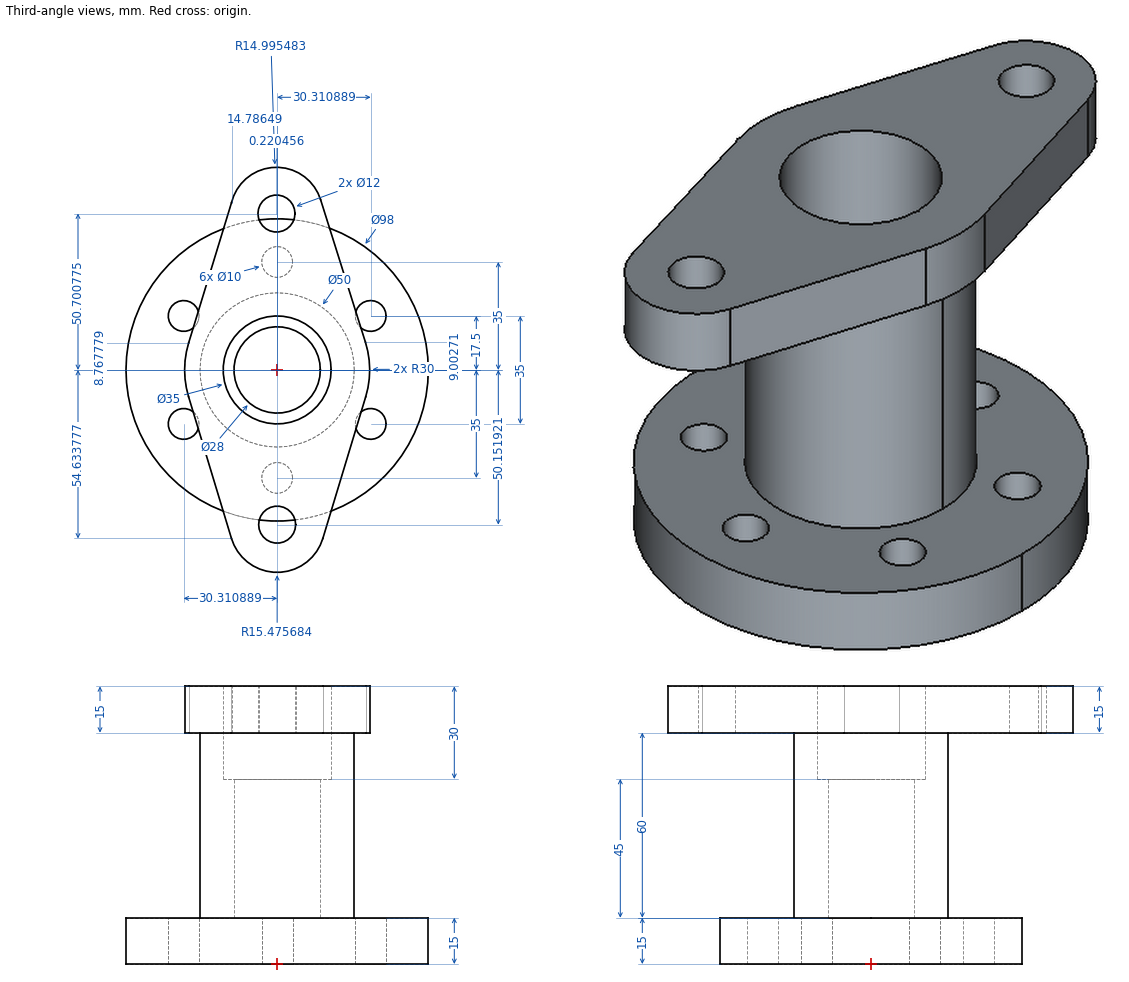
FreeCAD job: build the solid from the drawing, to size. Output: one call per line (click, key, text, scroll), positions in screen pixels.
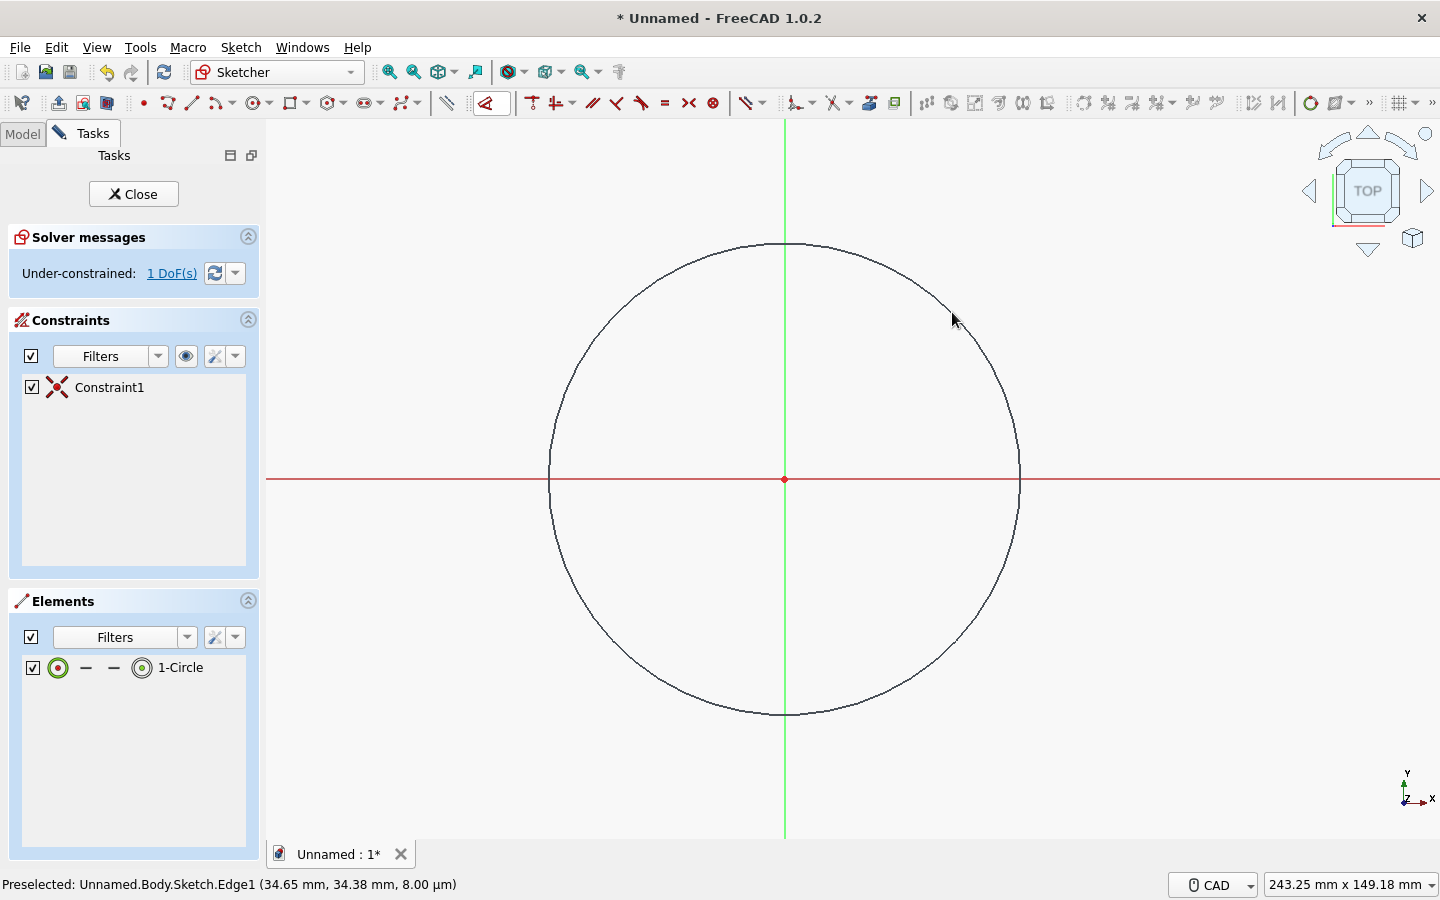
click(951, 312)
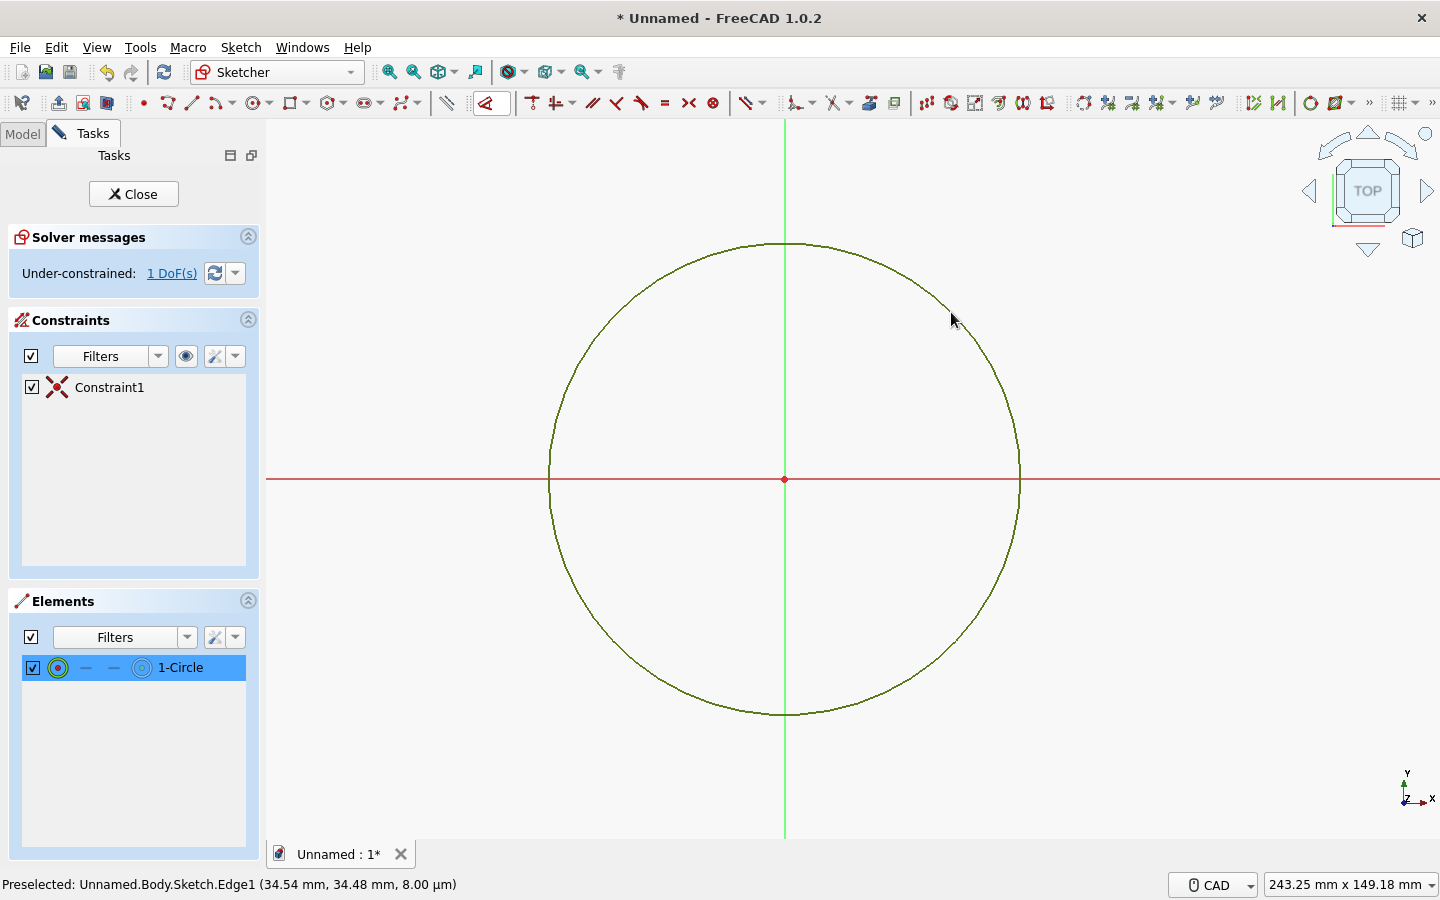
key(k)
key(o)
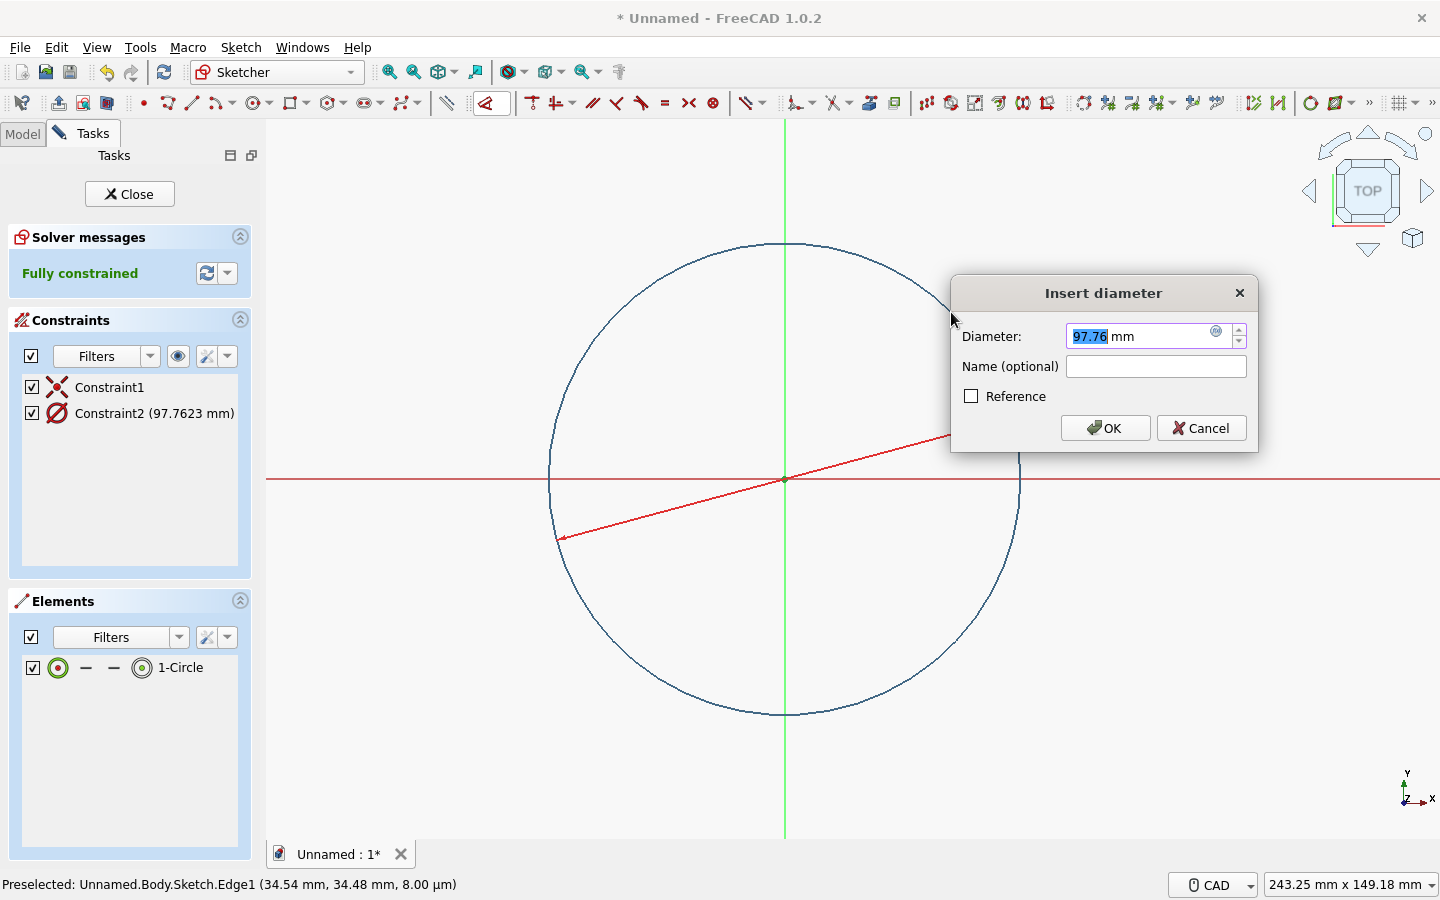
text(98)
key(Return)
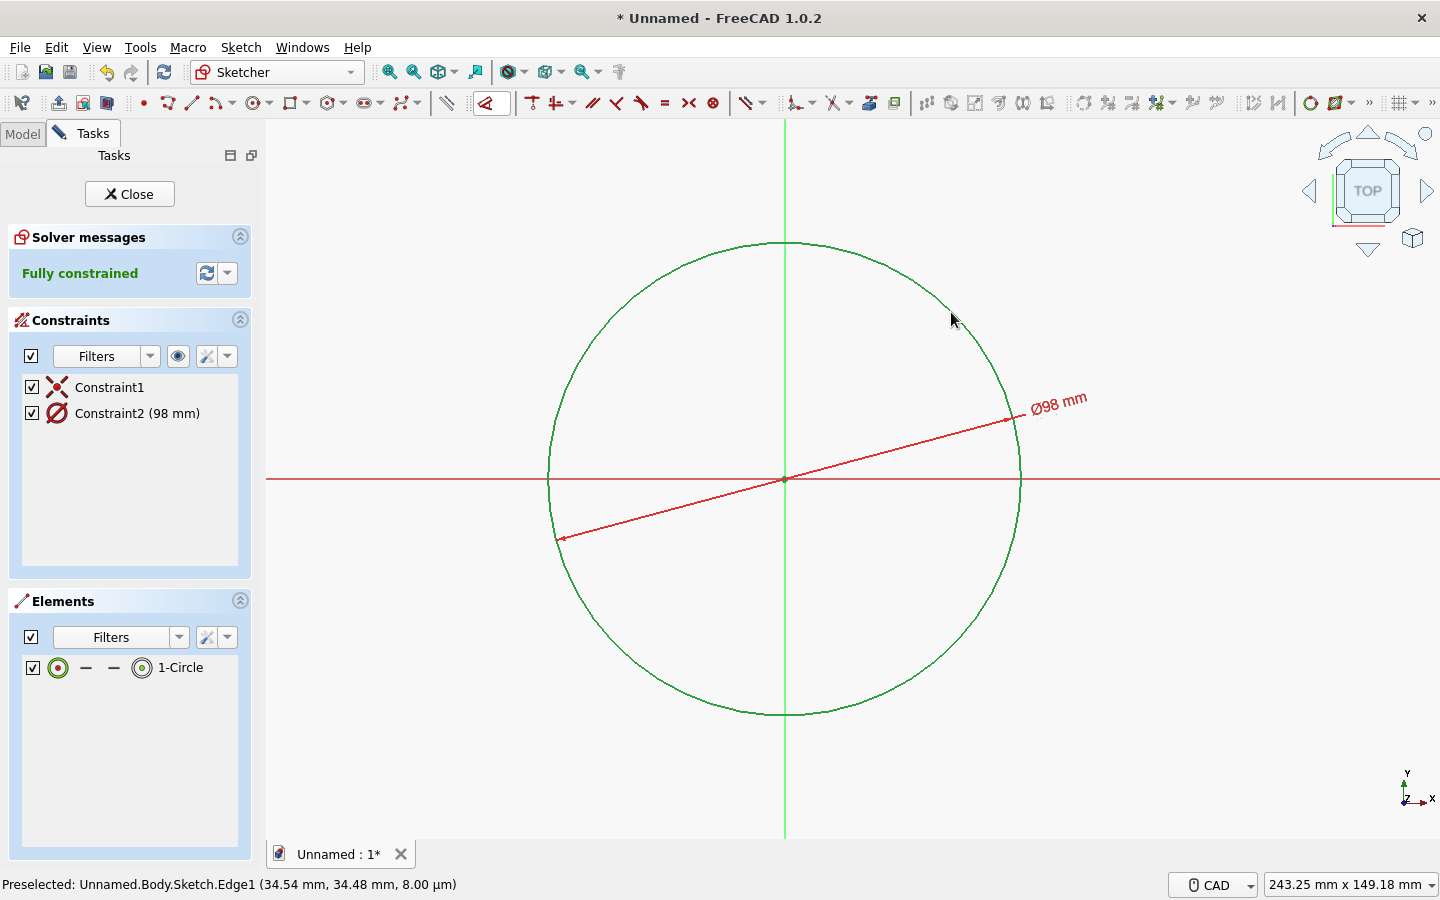
click(130, 194)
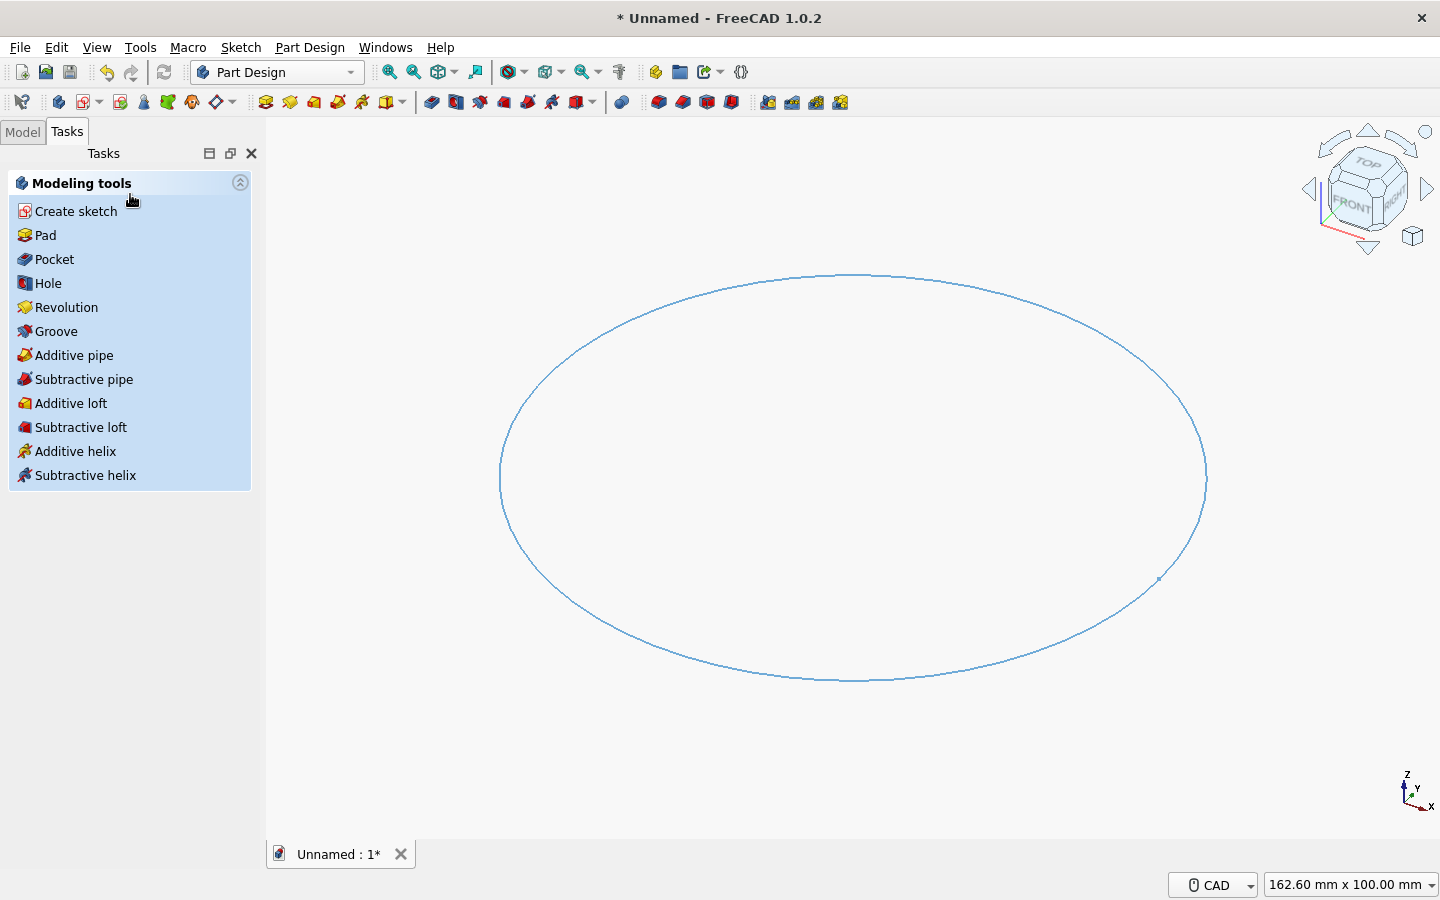
click(266, 102)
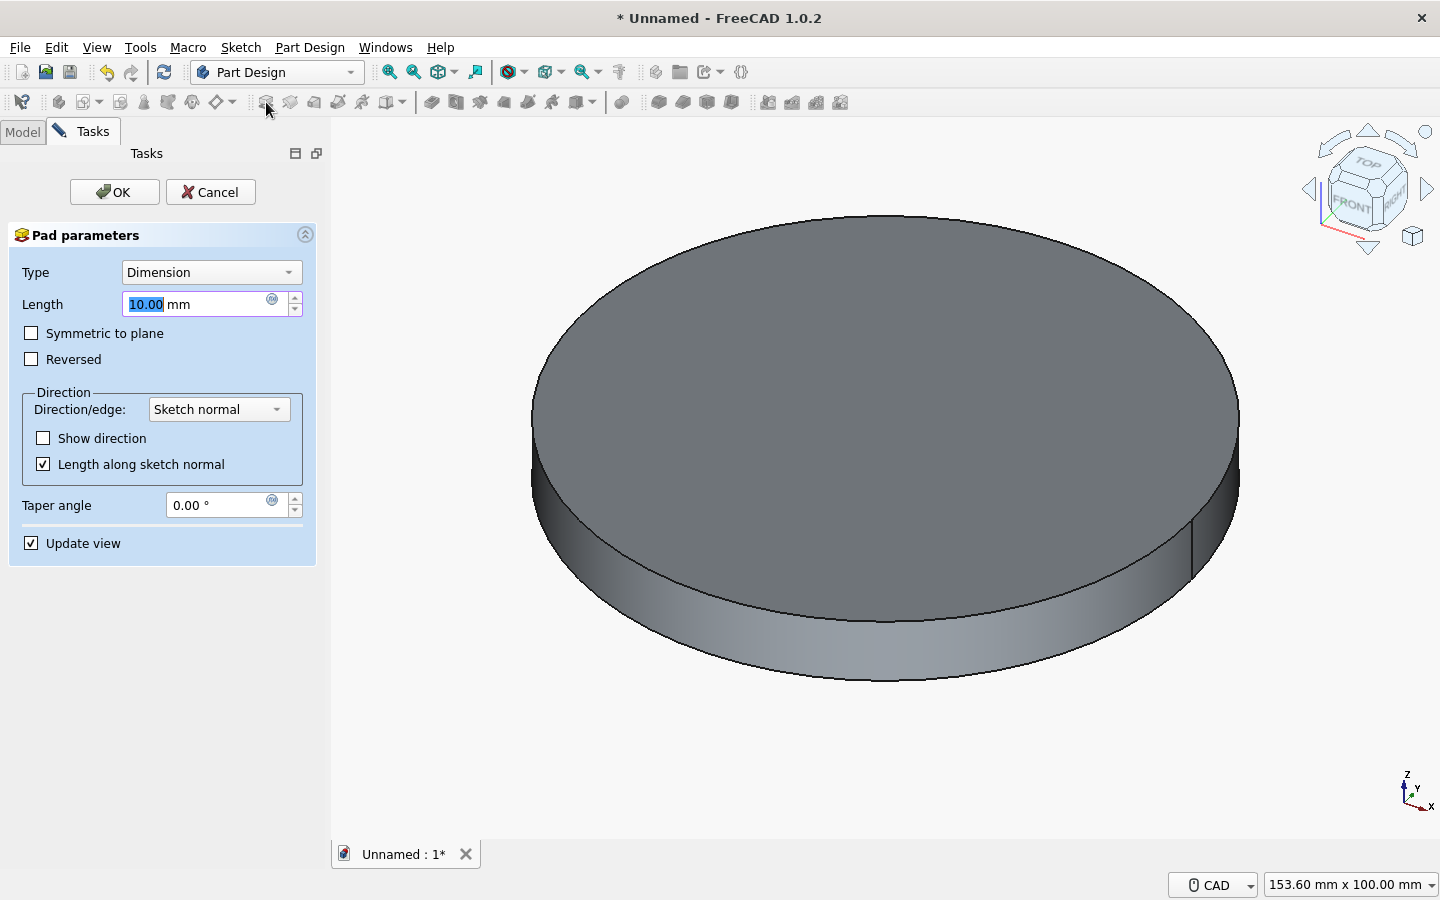
text(15)
key(Tab)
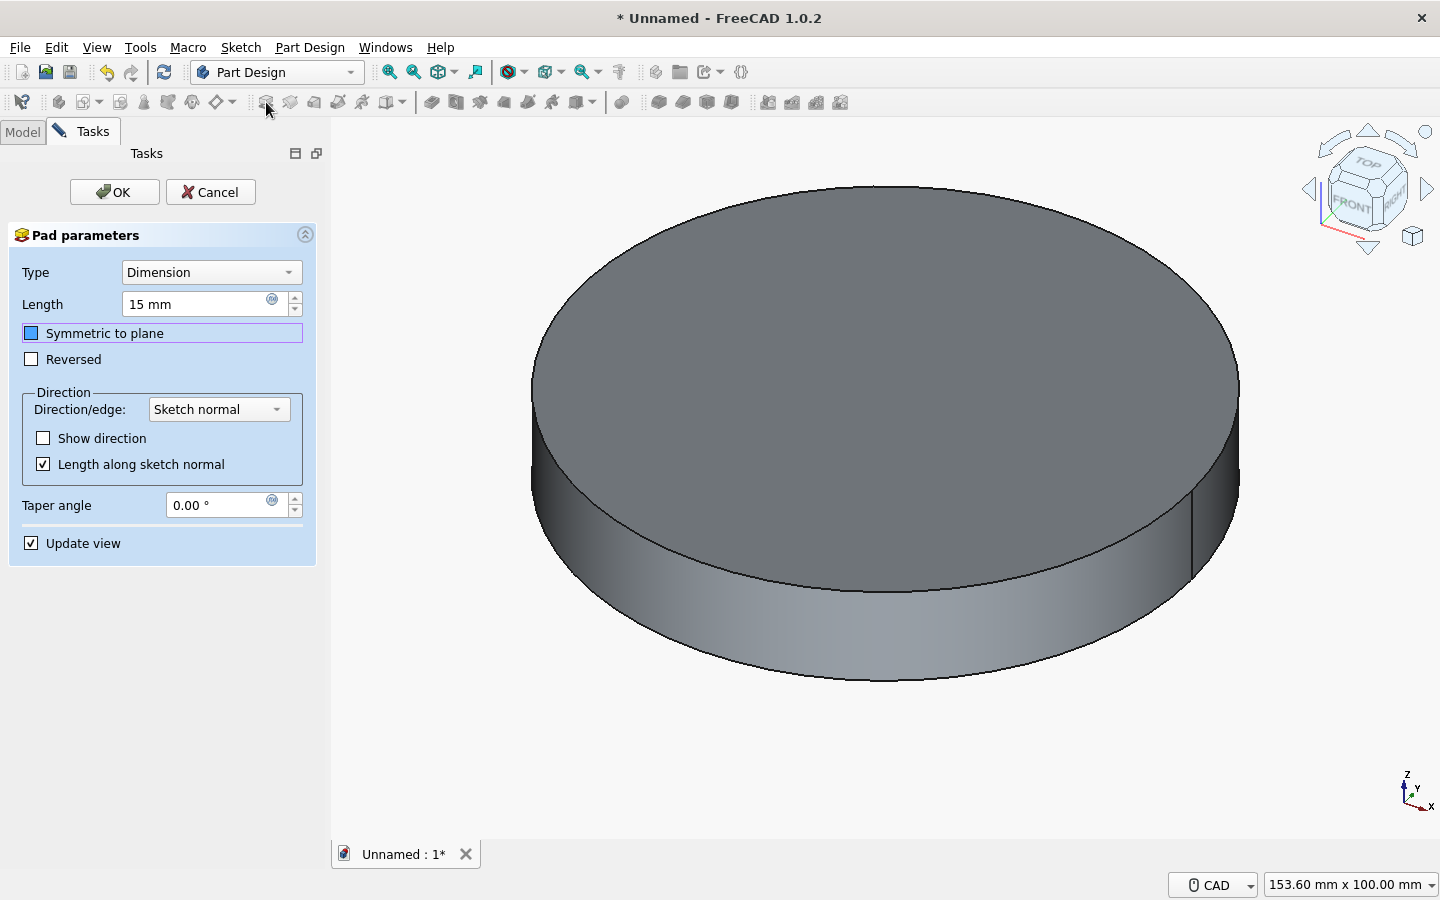
click(115, 192)